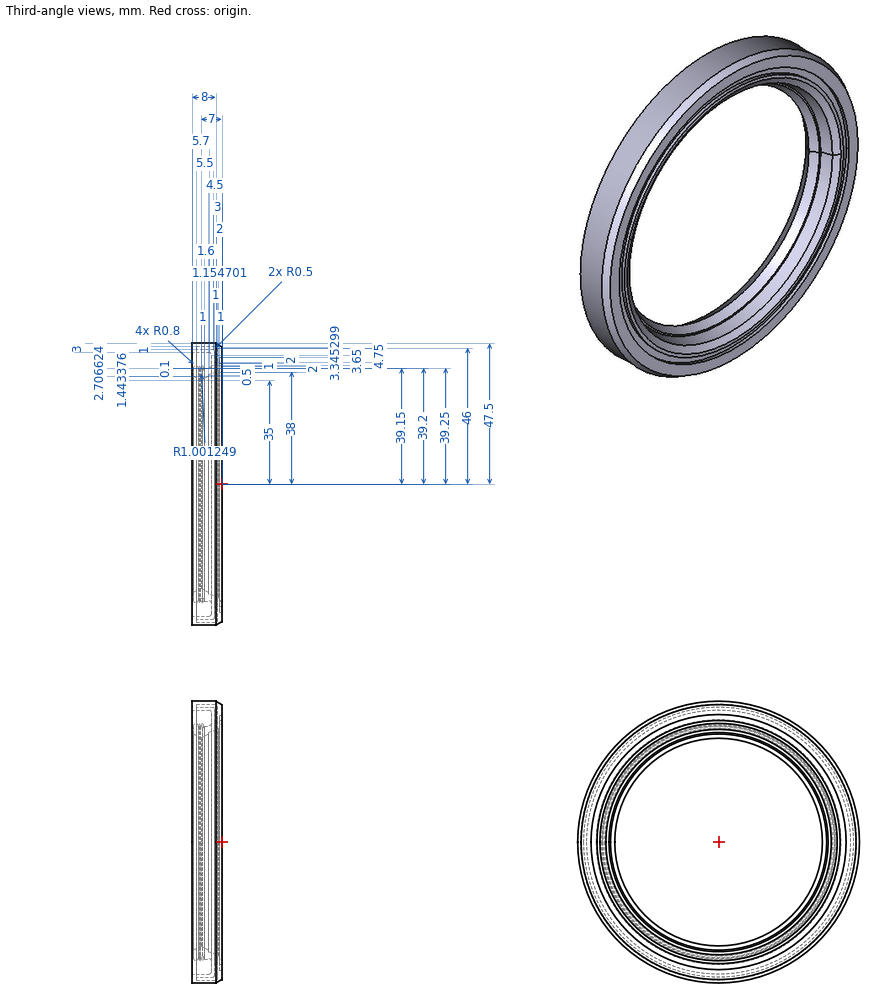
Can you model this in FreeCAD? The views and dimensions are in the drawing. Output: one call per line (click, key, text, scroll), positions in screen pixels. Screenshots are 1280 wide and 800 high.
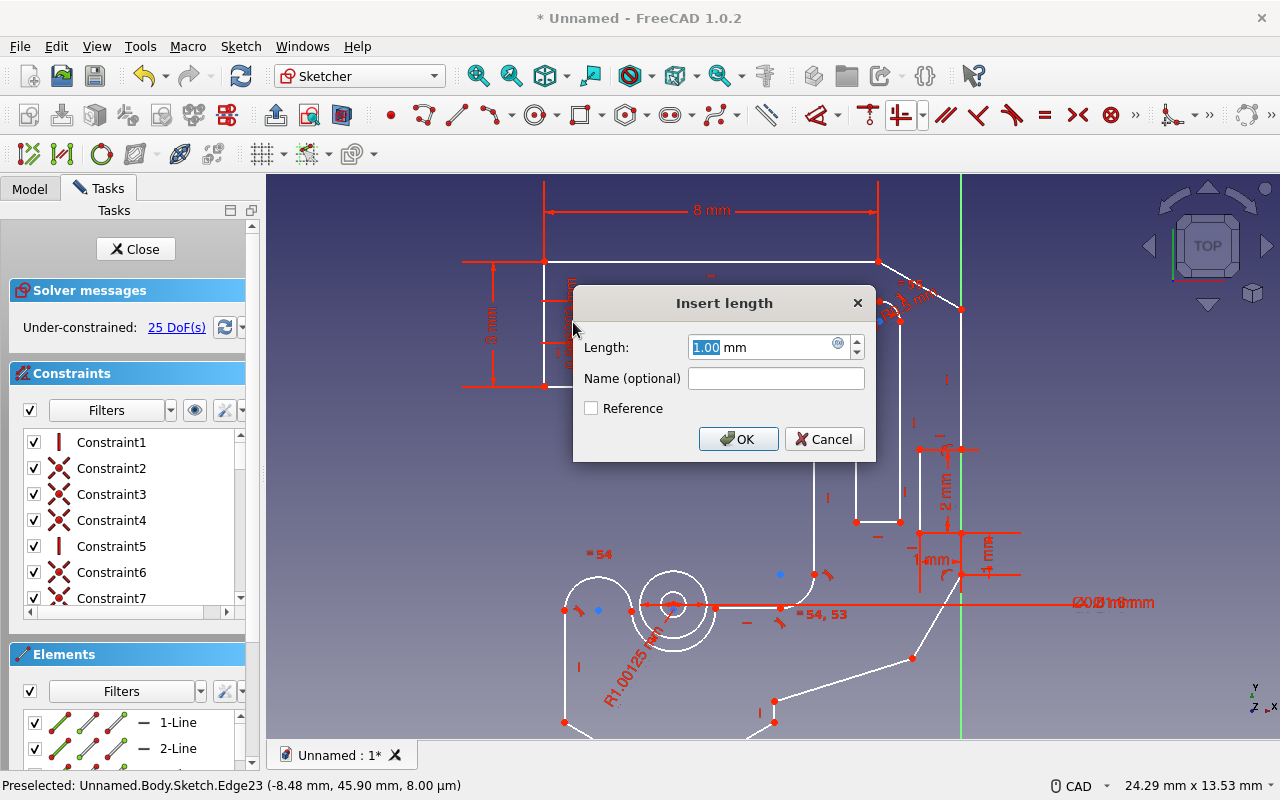
text(1)
key(Return)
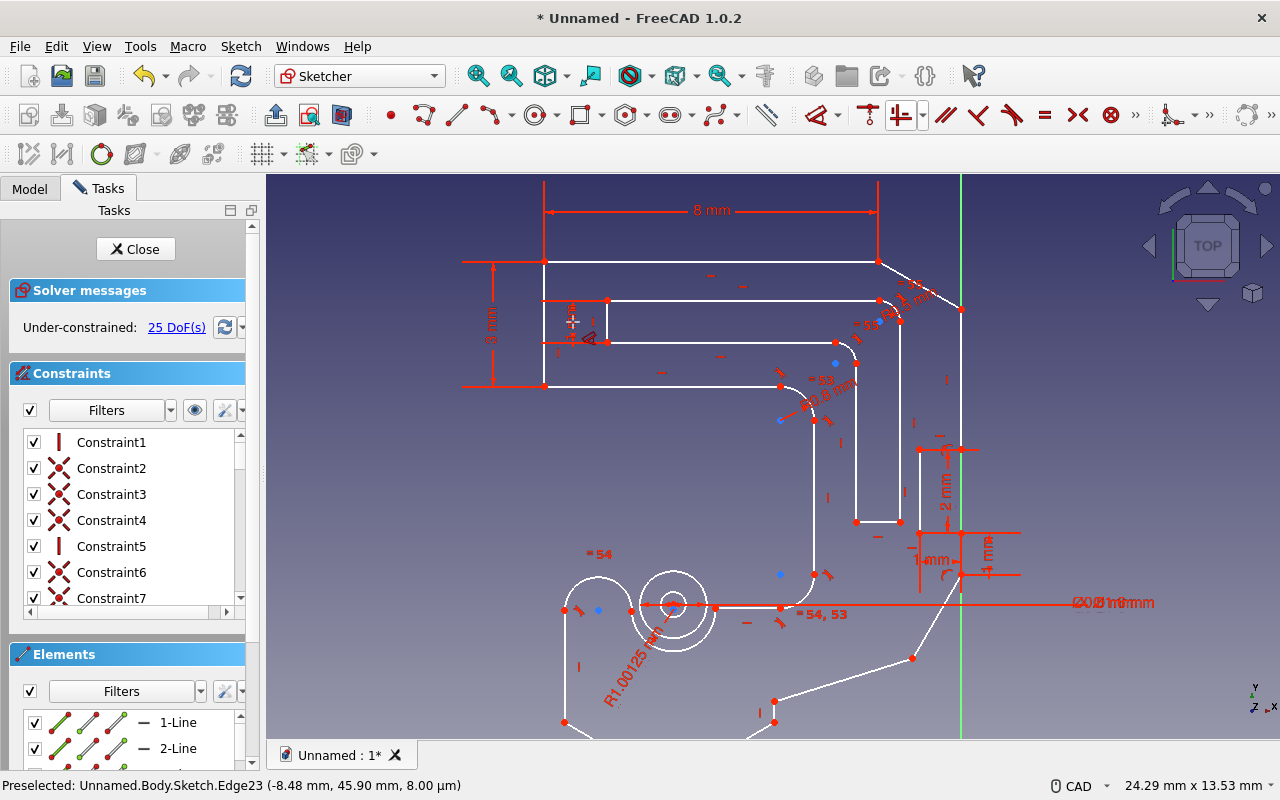
click(887, 522)
click(878, 464)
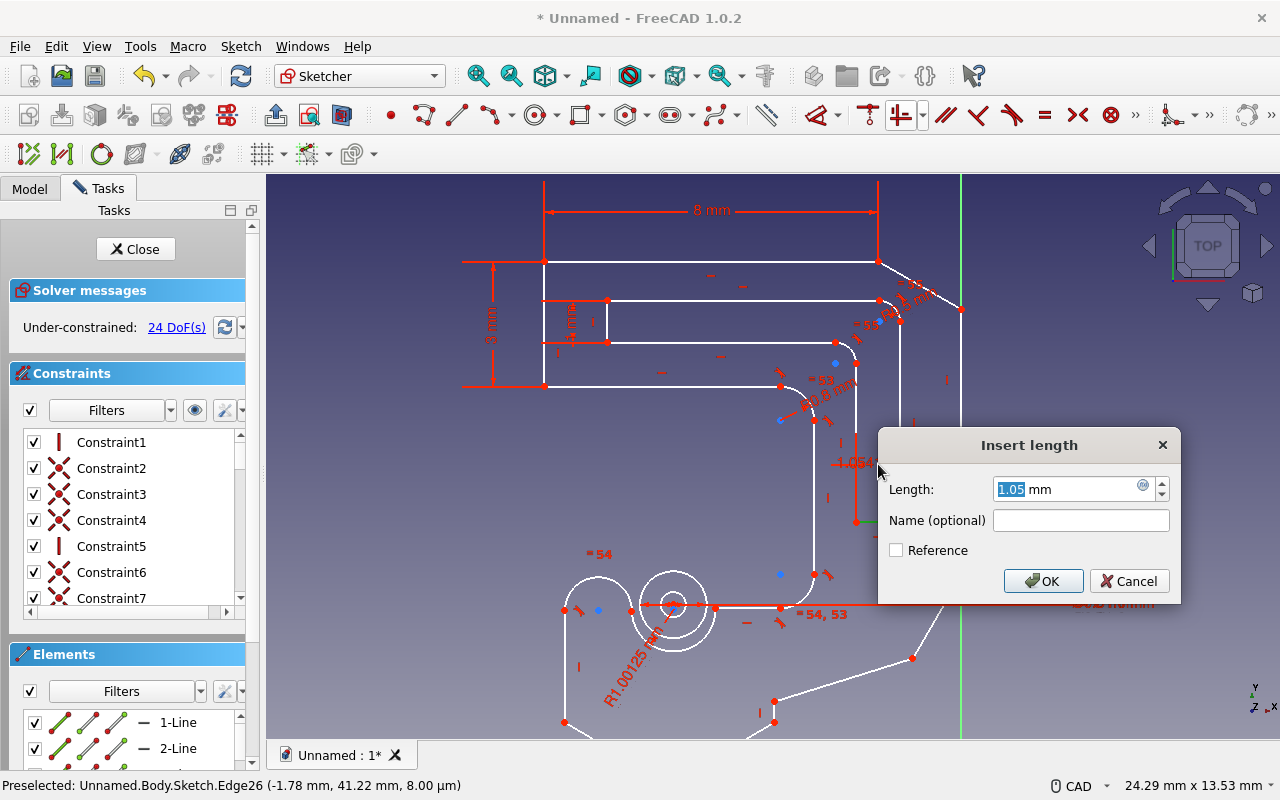
text(1)
key(Return)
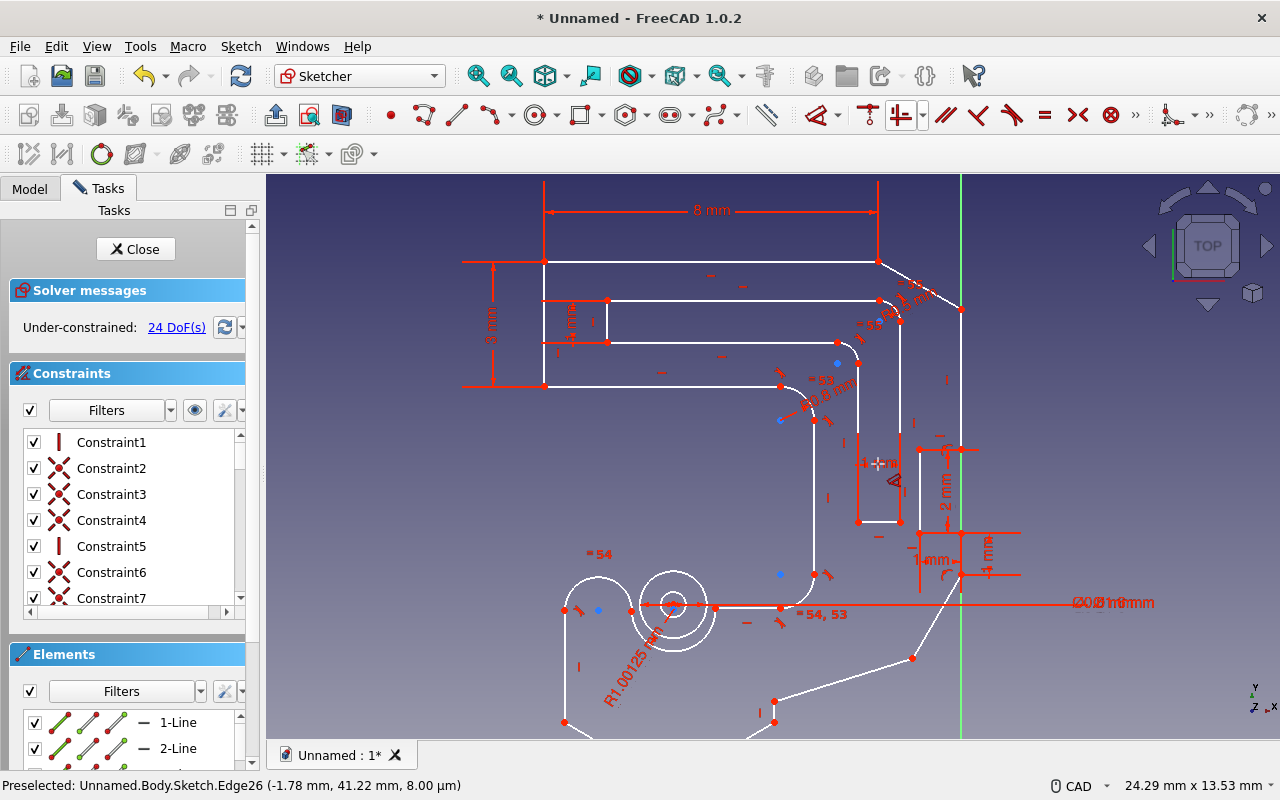
scroll(607, 325, down, 2)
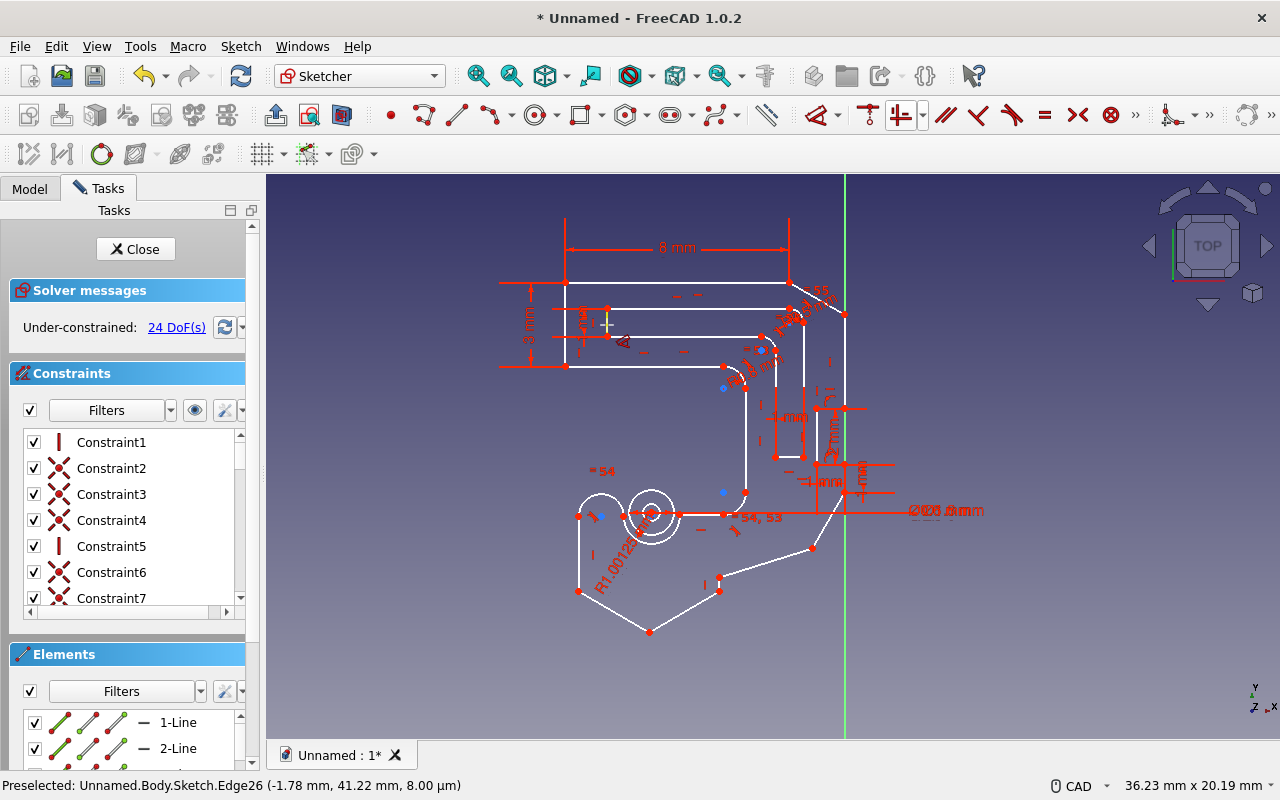
click(649, 633)
click(747, 599)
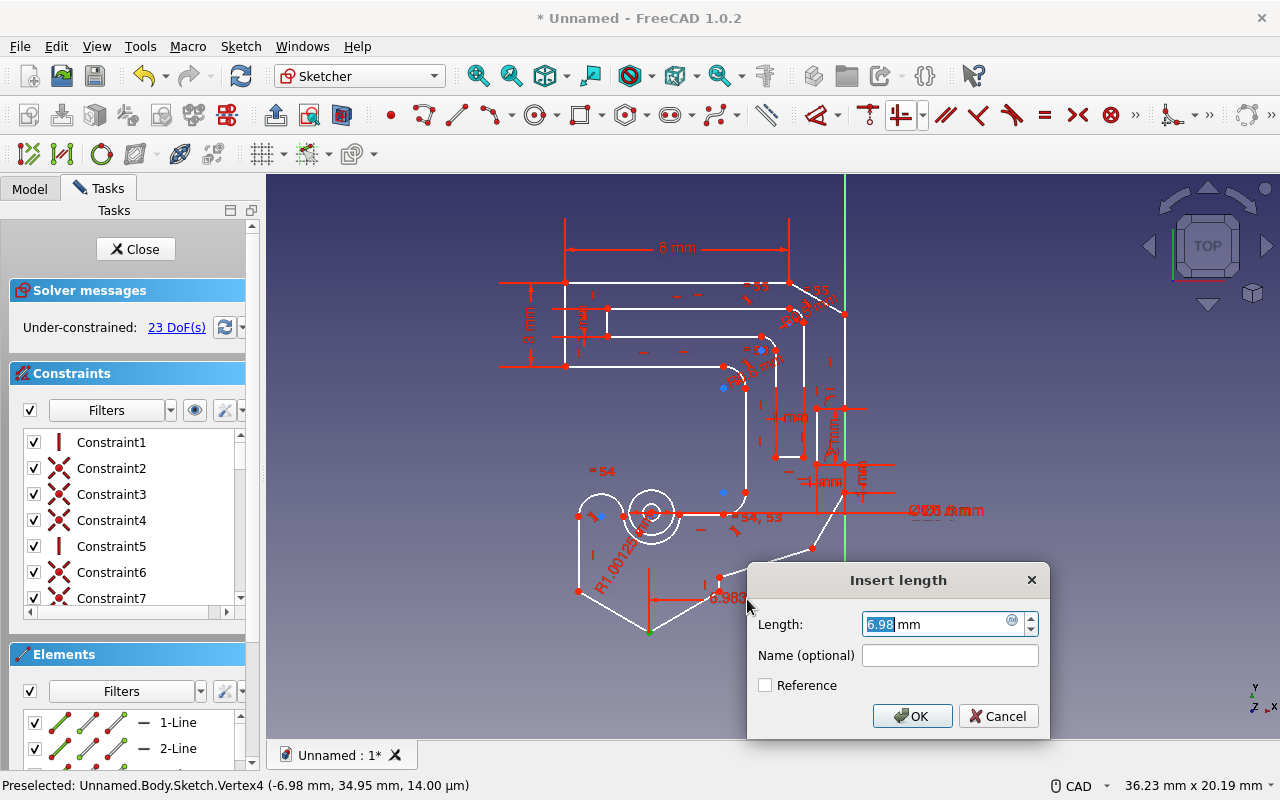
text(7)
key(Return)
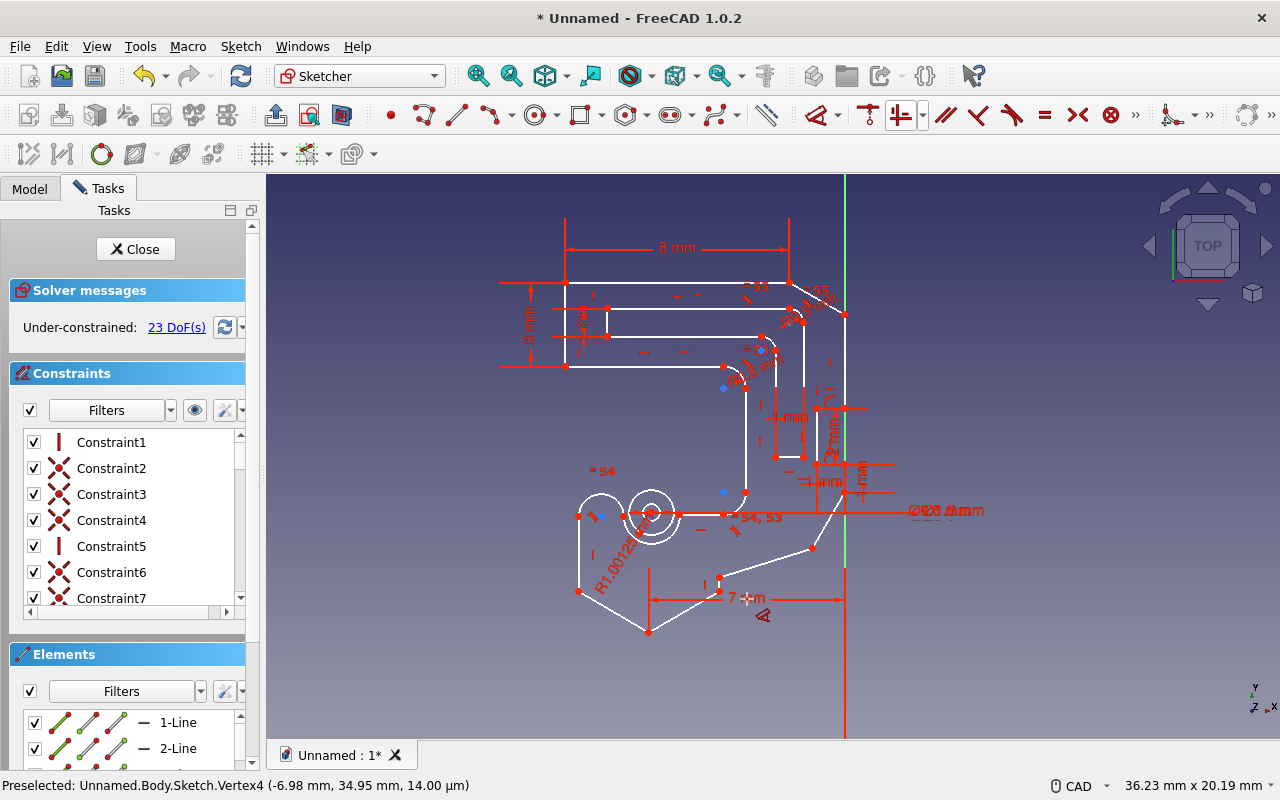
click(789, 283)
click(817, 249)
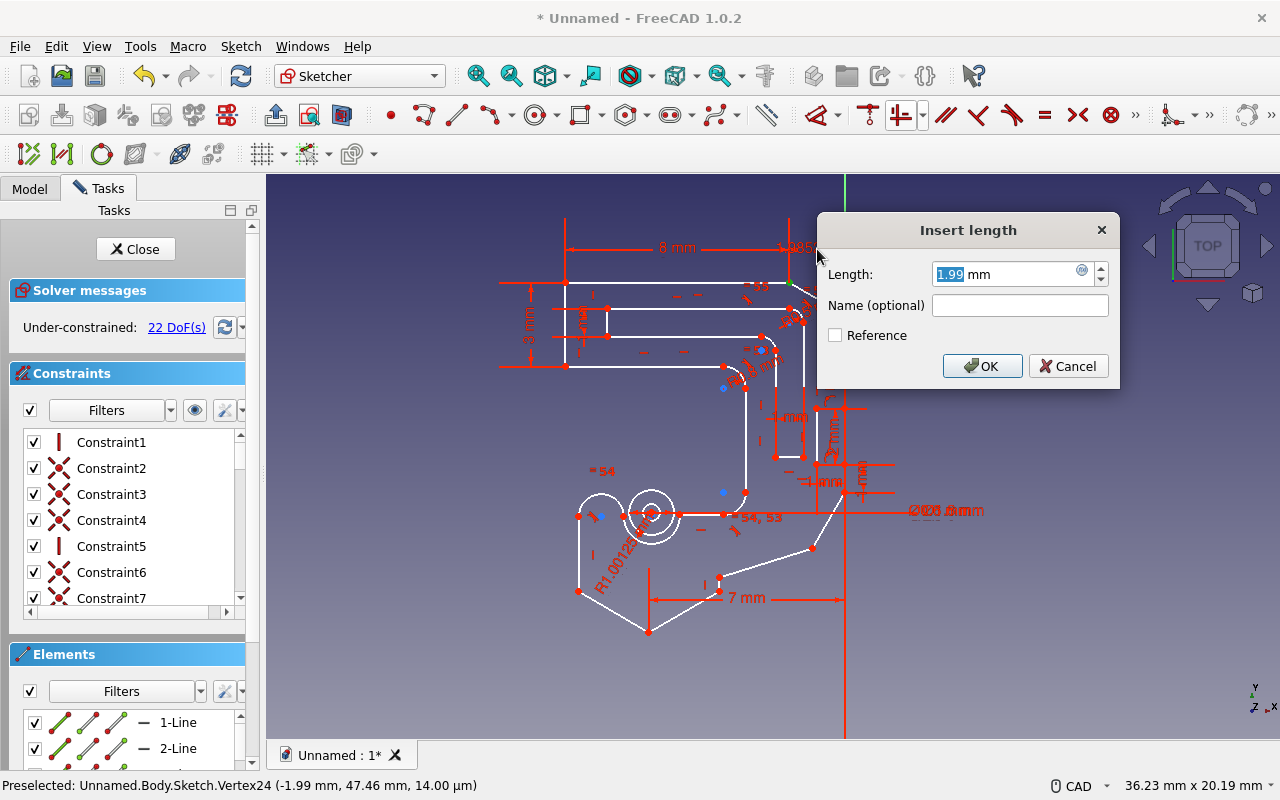
text(2)
key(Return)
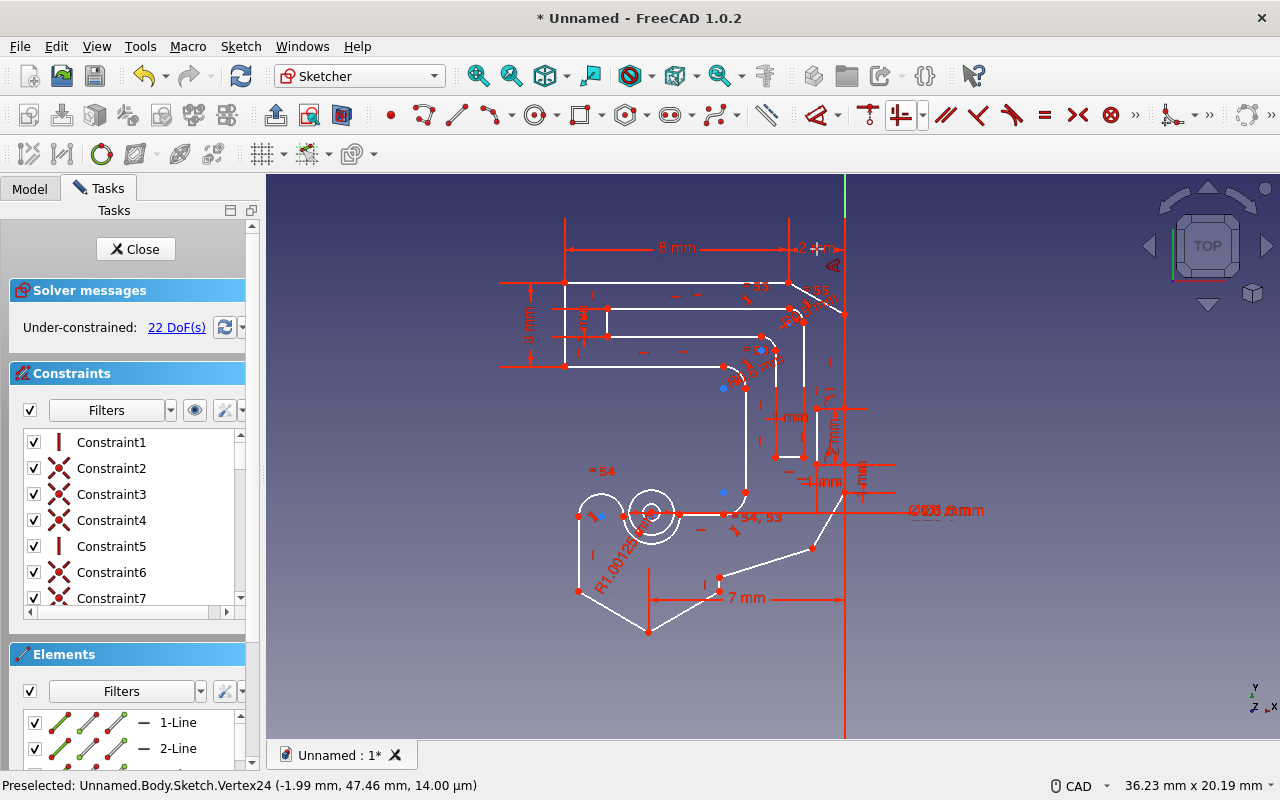
click(762, 337)
click(822, 279)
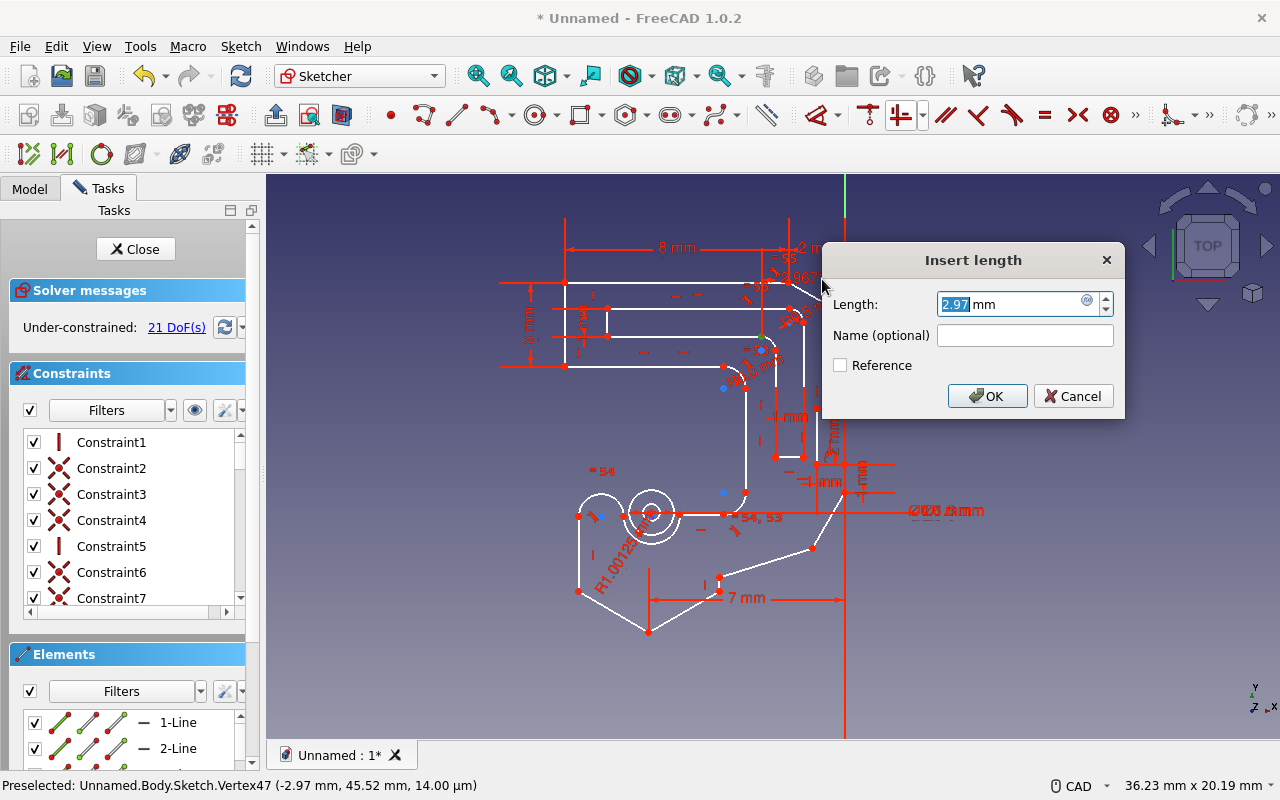
text(3)
key(Return)